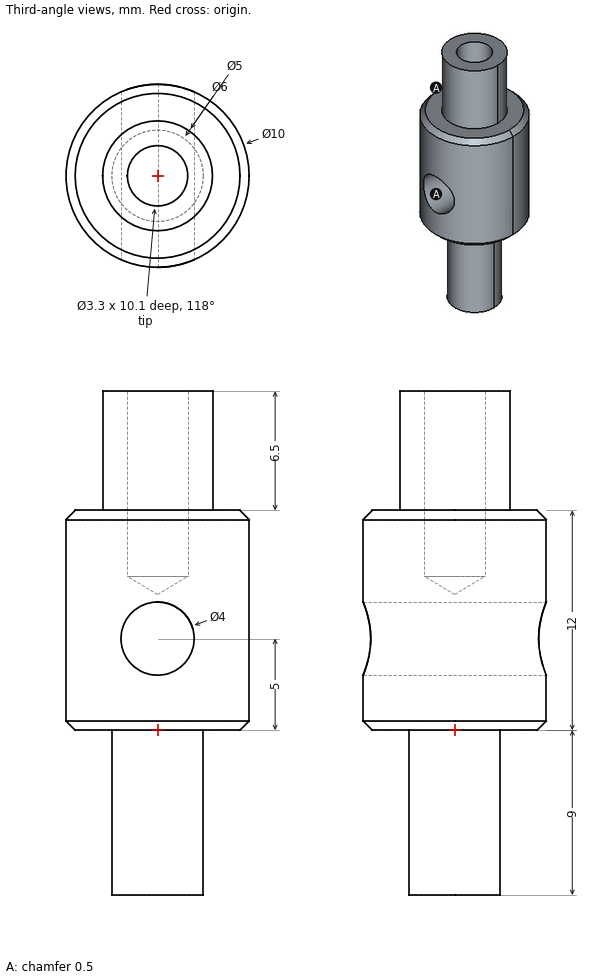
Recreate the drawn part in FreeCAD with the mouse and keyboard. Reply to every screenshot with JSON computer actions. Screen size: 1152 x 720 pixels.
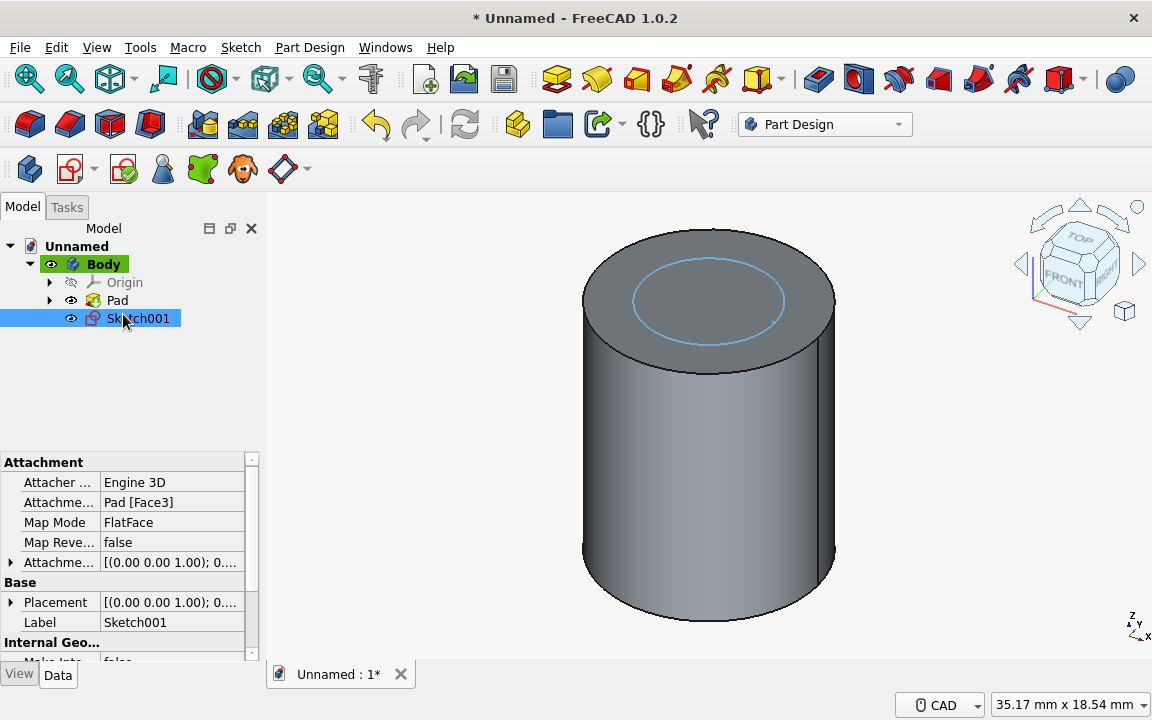
{"action": "left_click", "coordinate": [558, 80]}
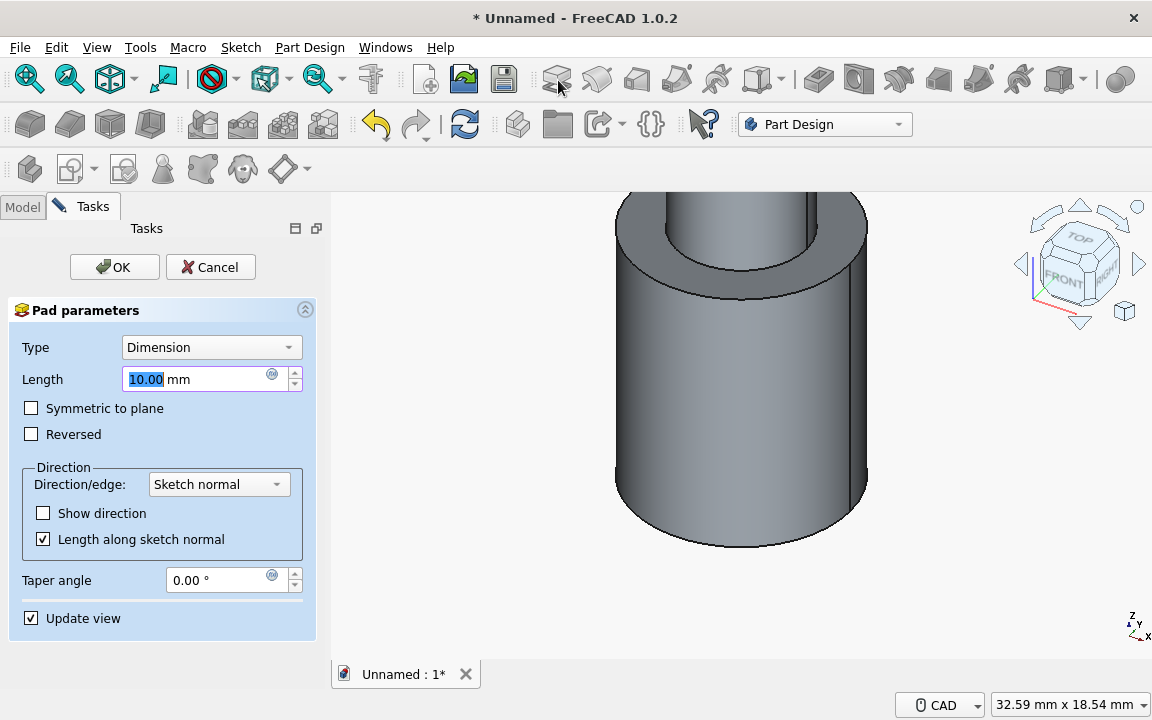
{"action": "type", "text": "6.5"}
{"action": "key", "text": "Tab"}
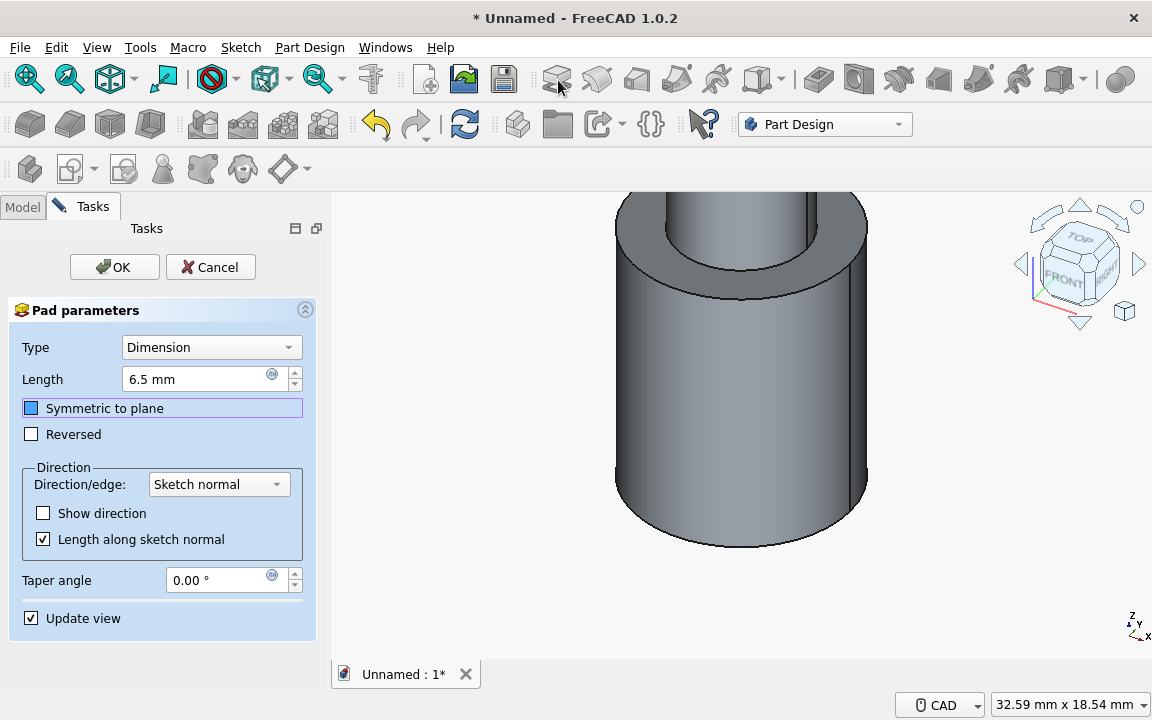
{"action": "left_click", "coordinate": [115, 267]}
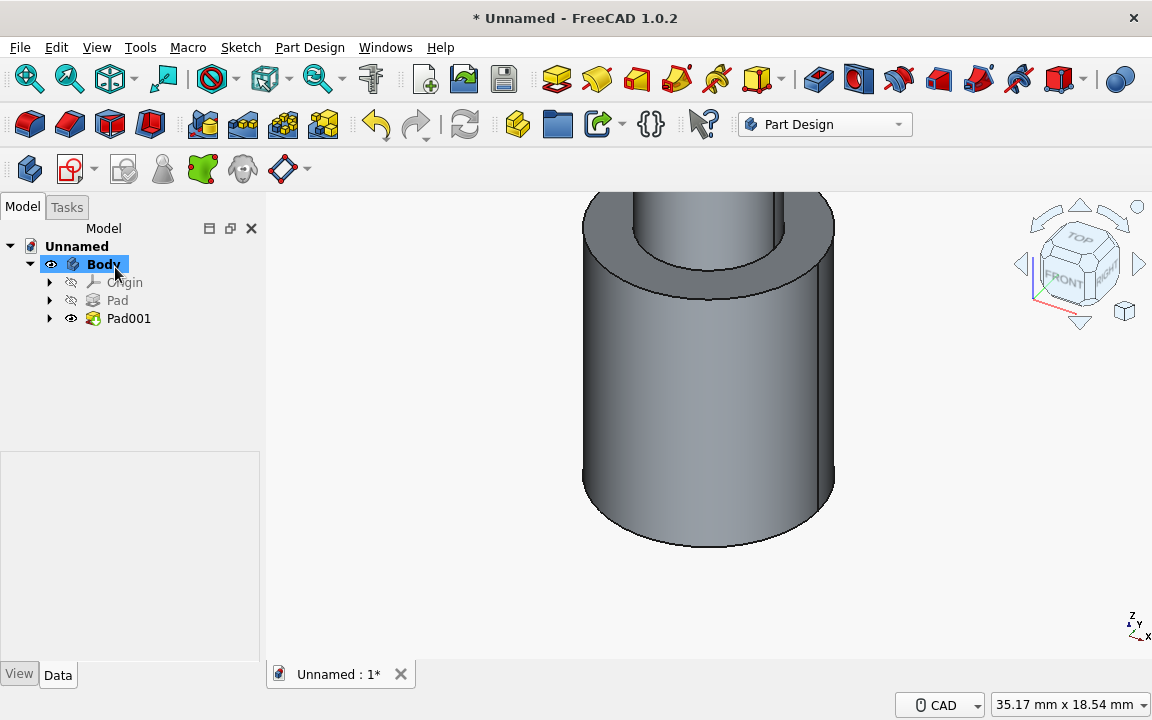
{"action": "key", "text": "v f"}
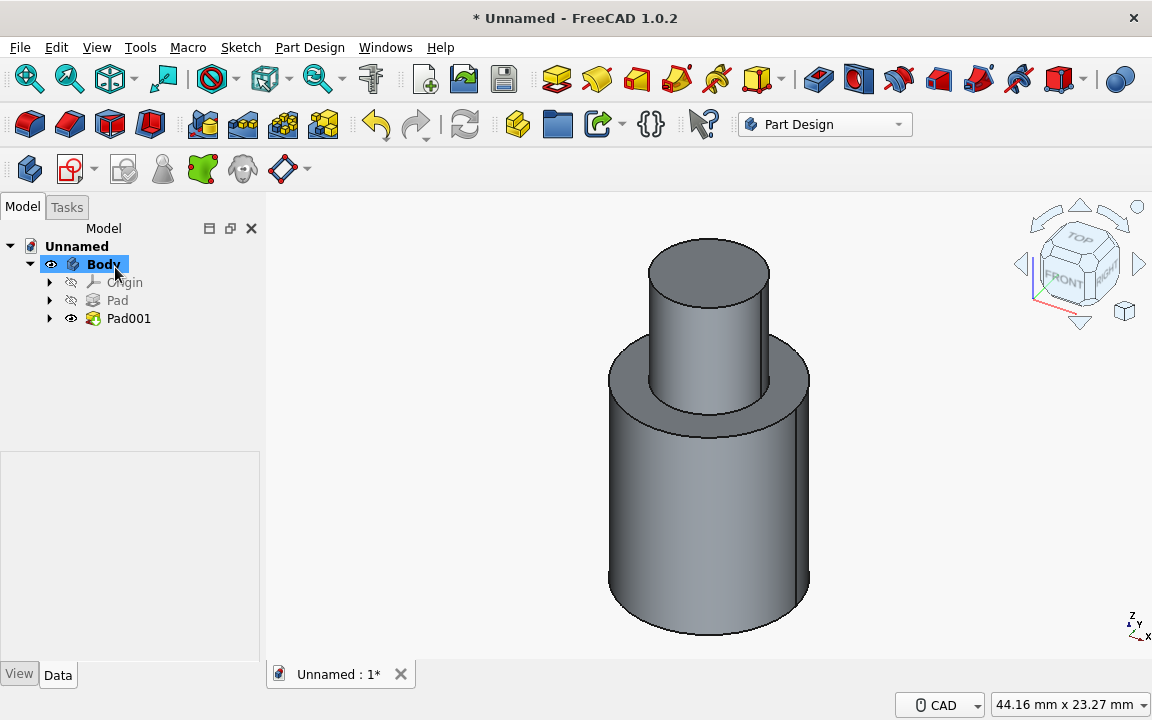
{"action": "left_click", "coordinate": [709, 272]}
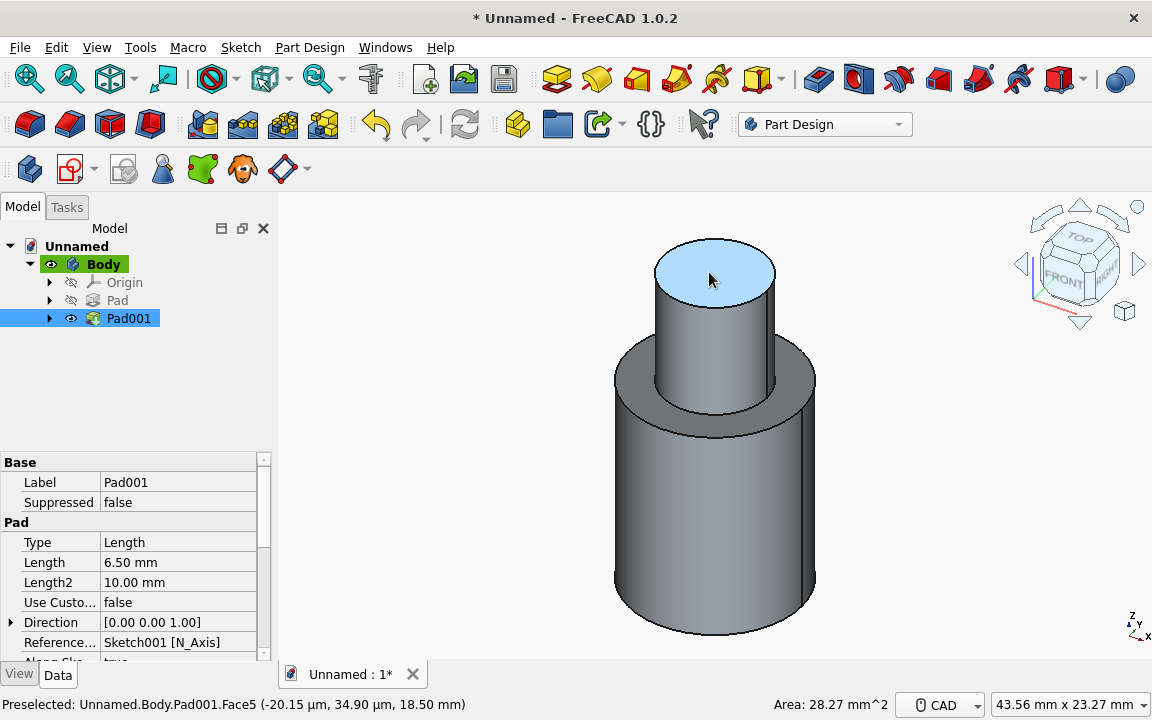
{"action": "left_click", "coordinate": [70, 170]}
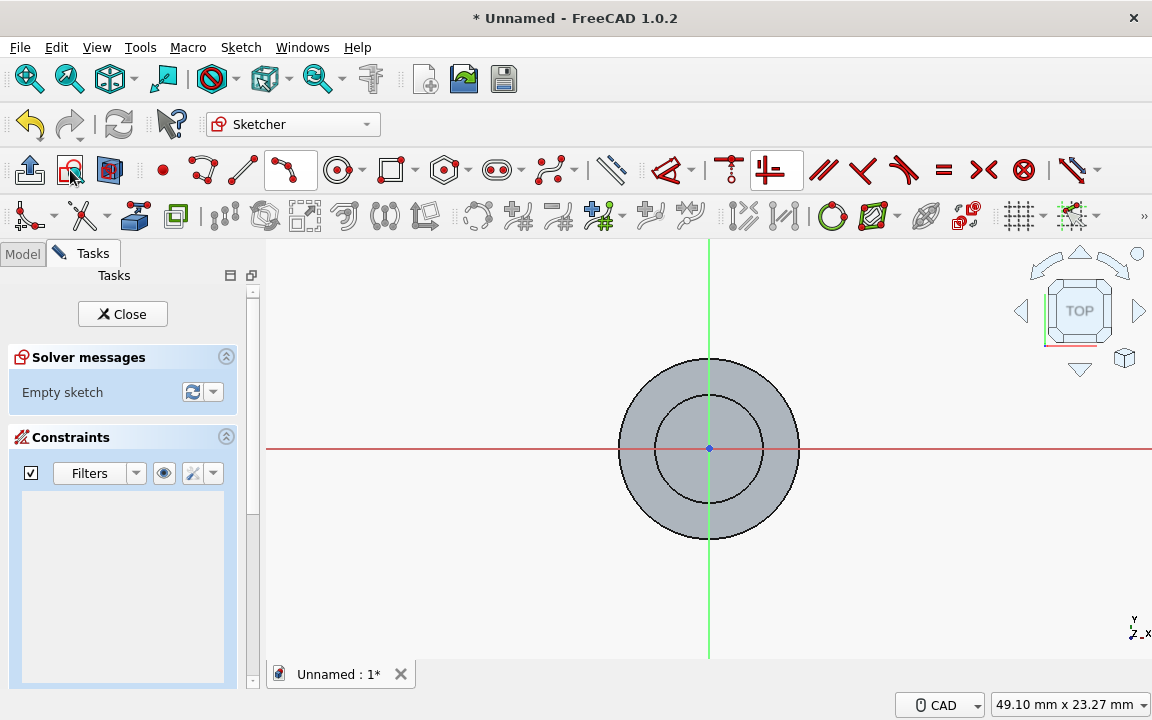
{"action": "scroll", "coordinate": [731, 449], "scroll_direction": "up", "scroll_amount": 7}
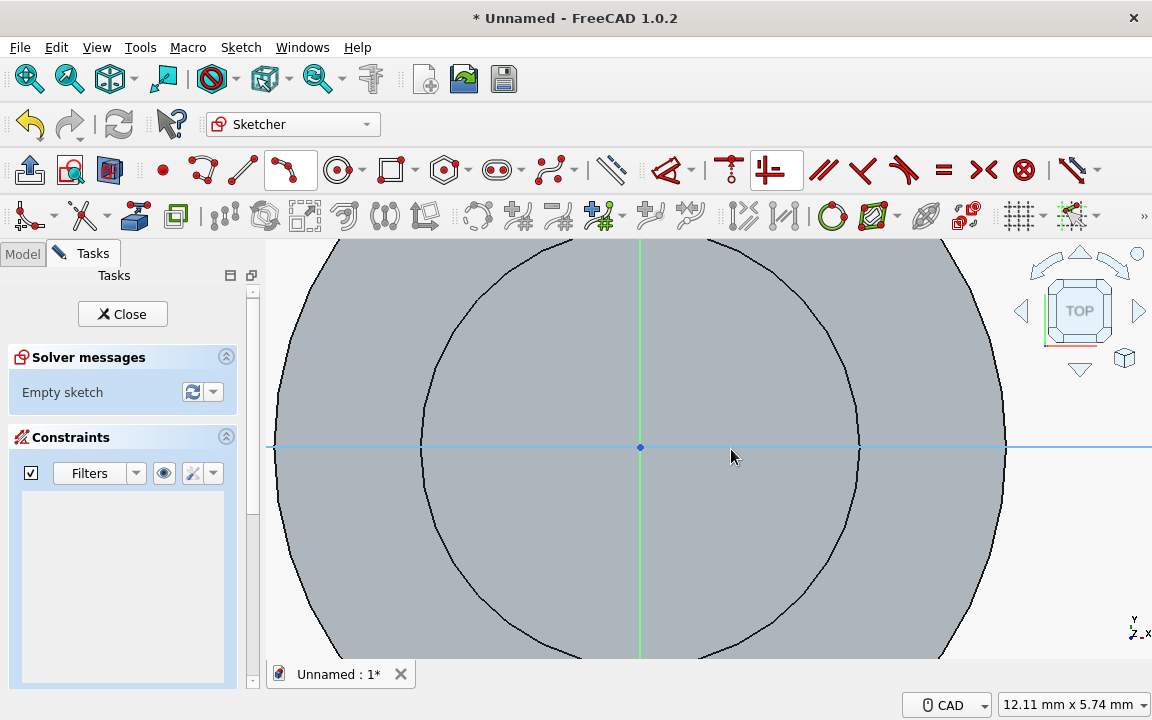
{"action": "key", "text": "g c"}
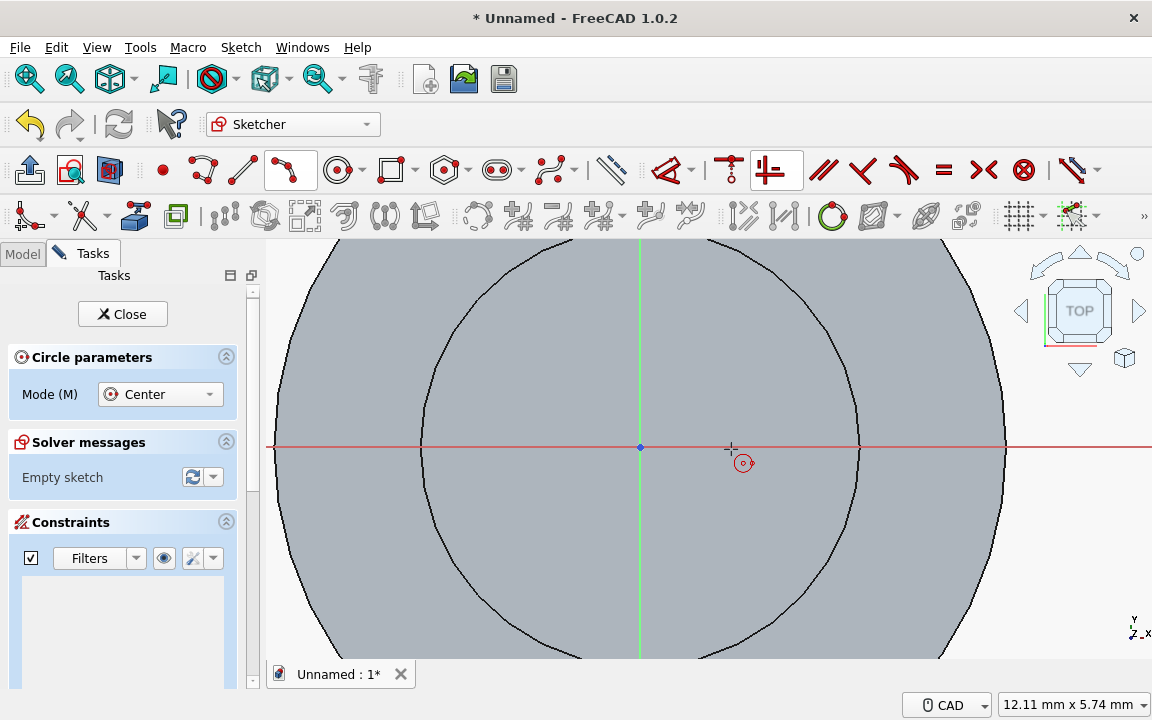
{"action": "left_click", "coordinate": [640, 447]}
{"action": "left_click", "coordinate": [726, 362]}
{"action": "key", "text": "Escape"}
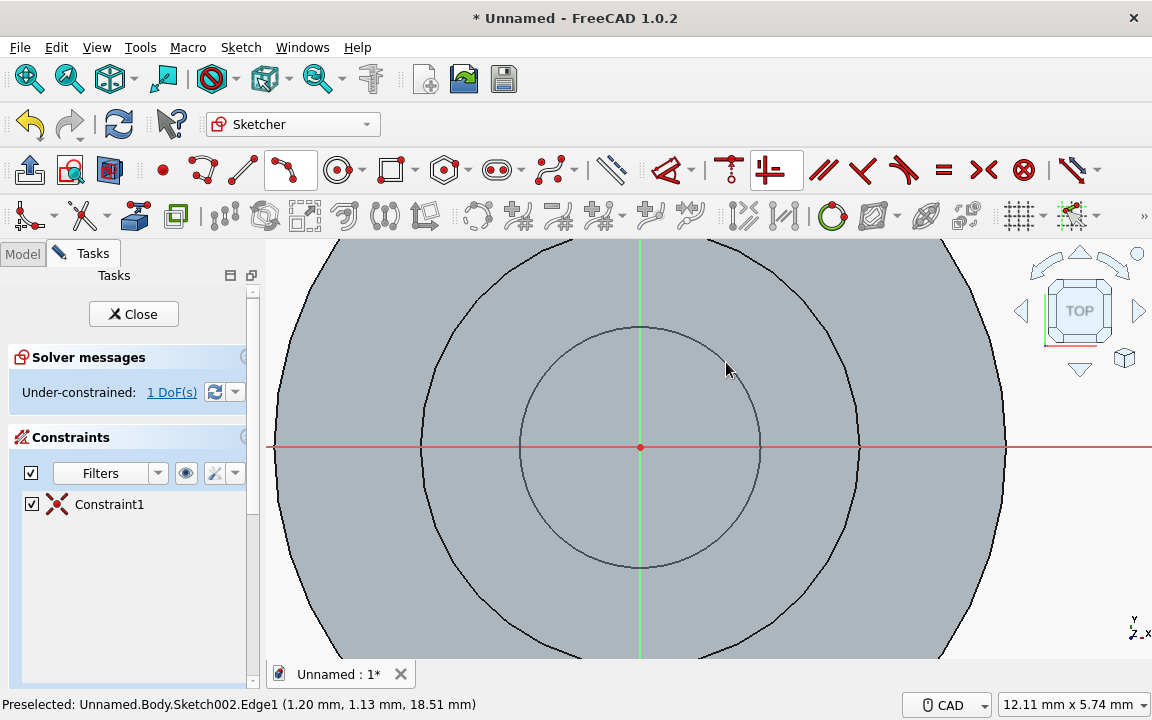
{"action": "left_click", "coordinate": [666, 170]}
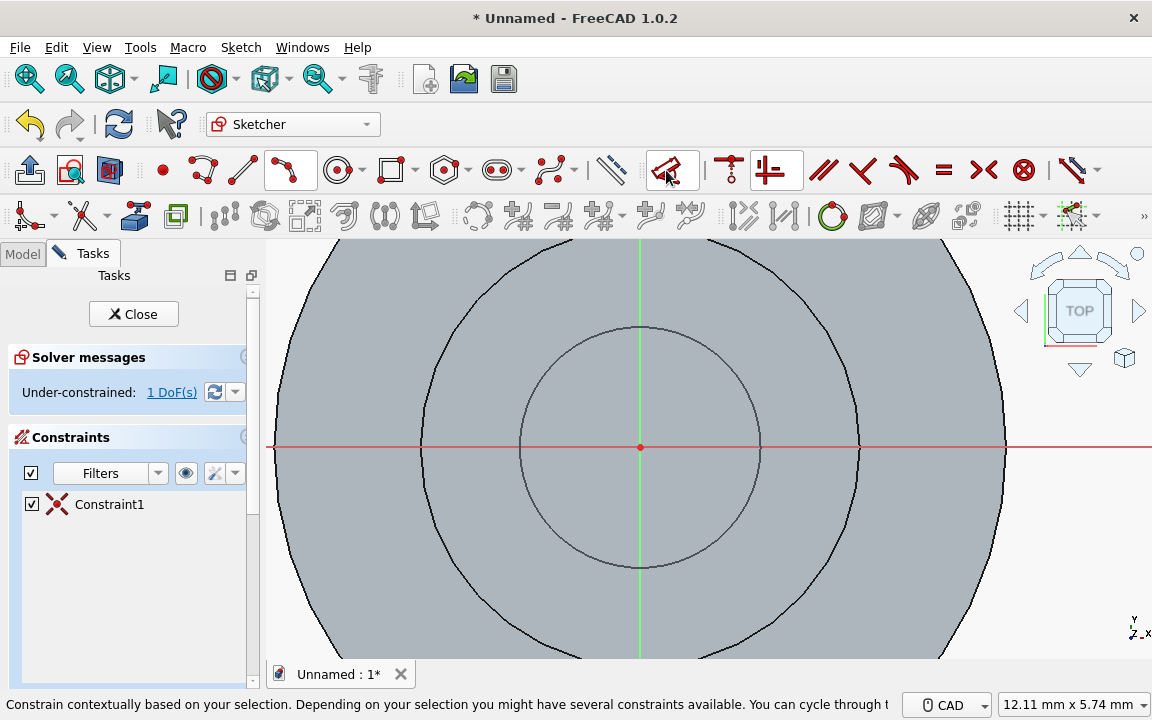
{"action": "left_click", "coordinate": [725, 362]}
{"action": "left_click", "coordinate": [748, 339]}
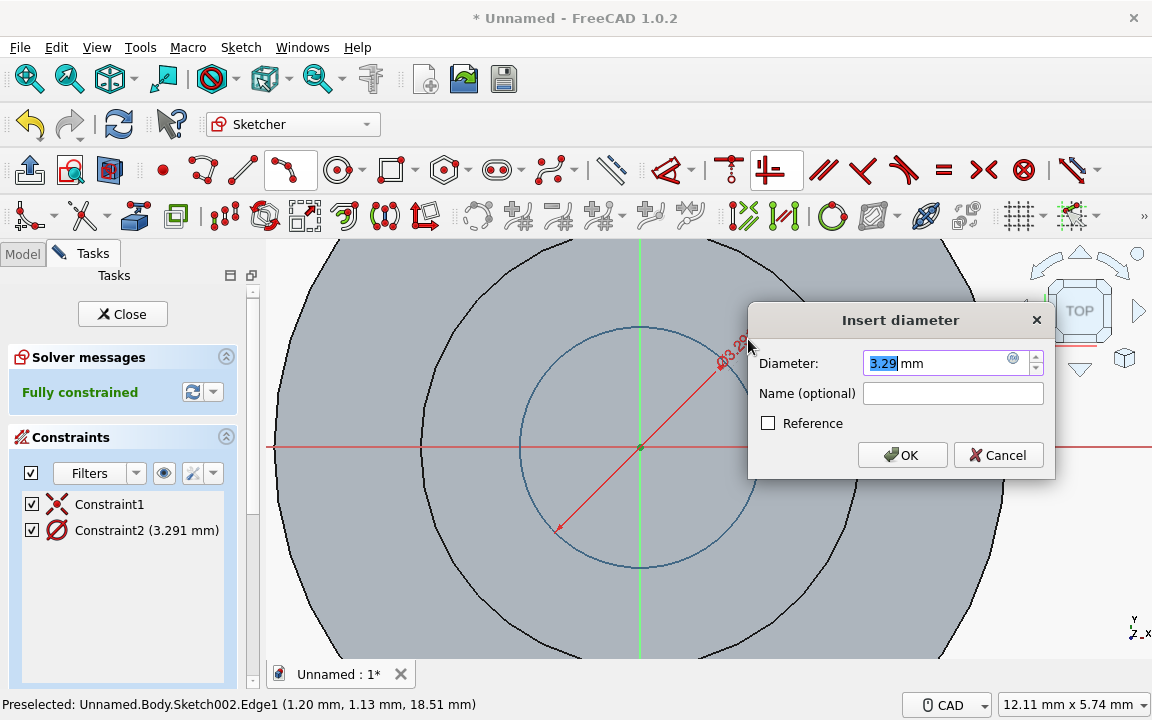
{"action": "type", "text": "3.3"}
{"action": "key", "text": "Return"}
{"action": "key", "text": "Escape"}